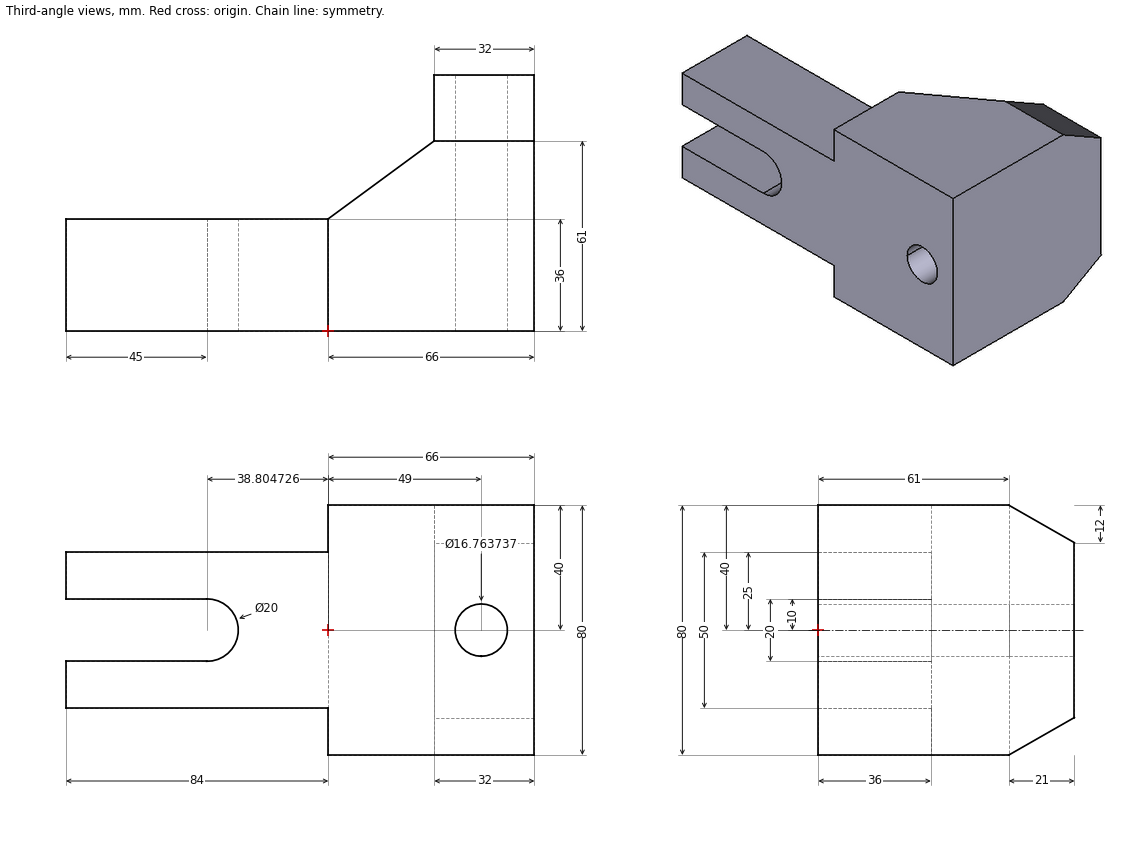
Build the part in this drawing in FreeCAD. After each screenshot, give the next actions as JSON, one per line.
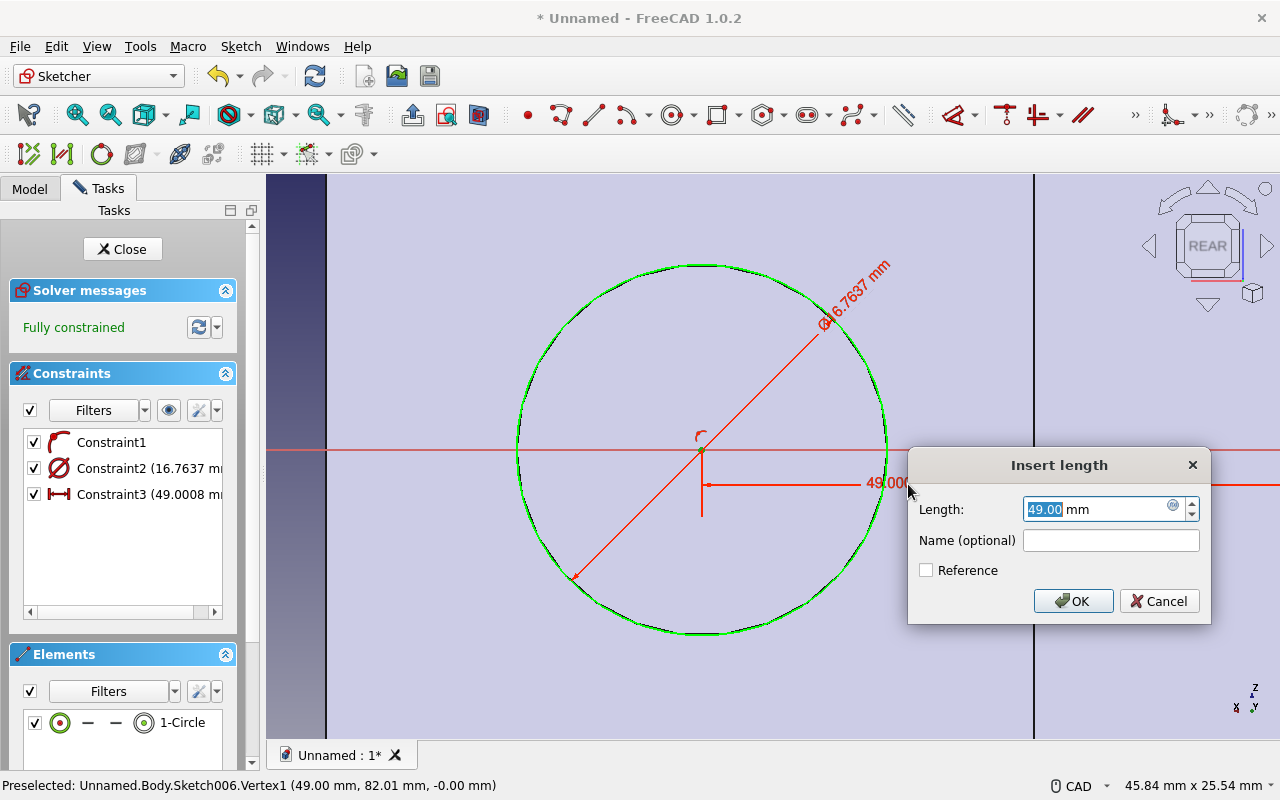
{"action": "type", "text": "49"}
{"action": "key", "text": "Return"}
{"action": "key", "text": "Escape"}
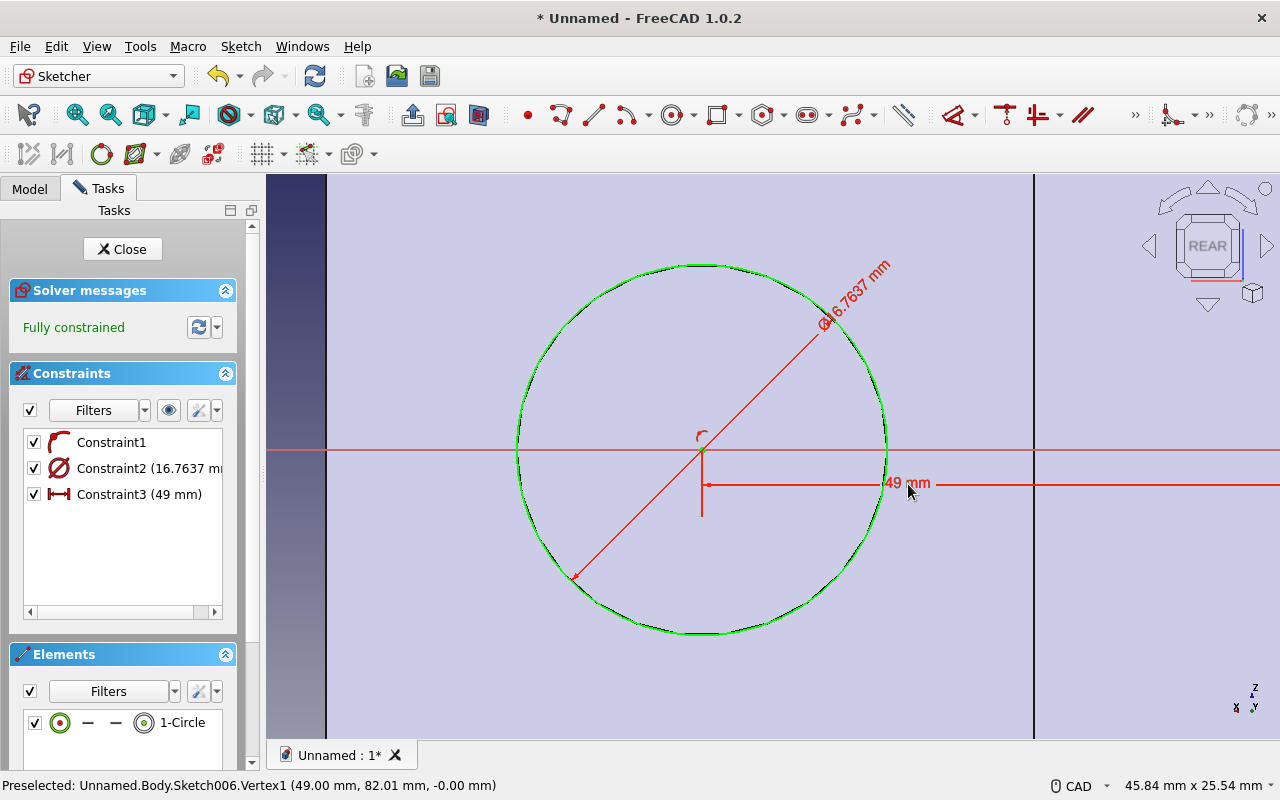
{"action": "left_click", "coordinate": [123, 249]}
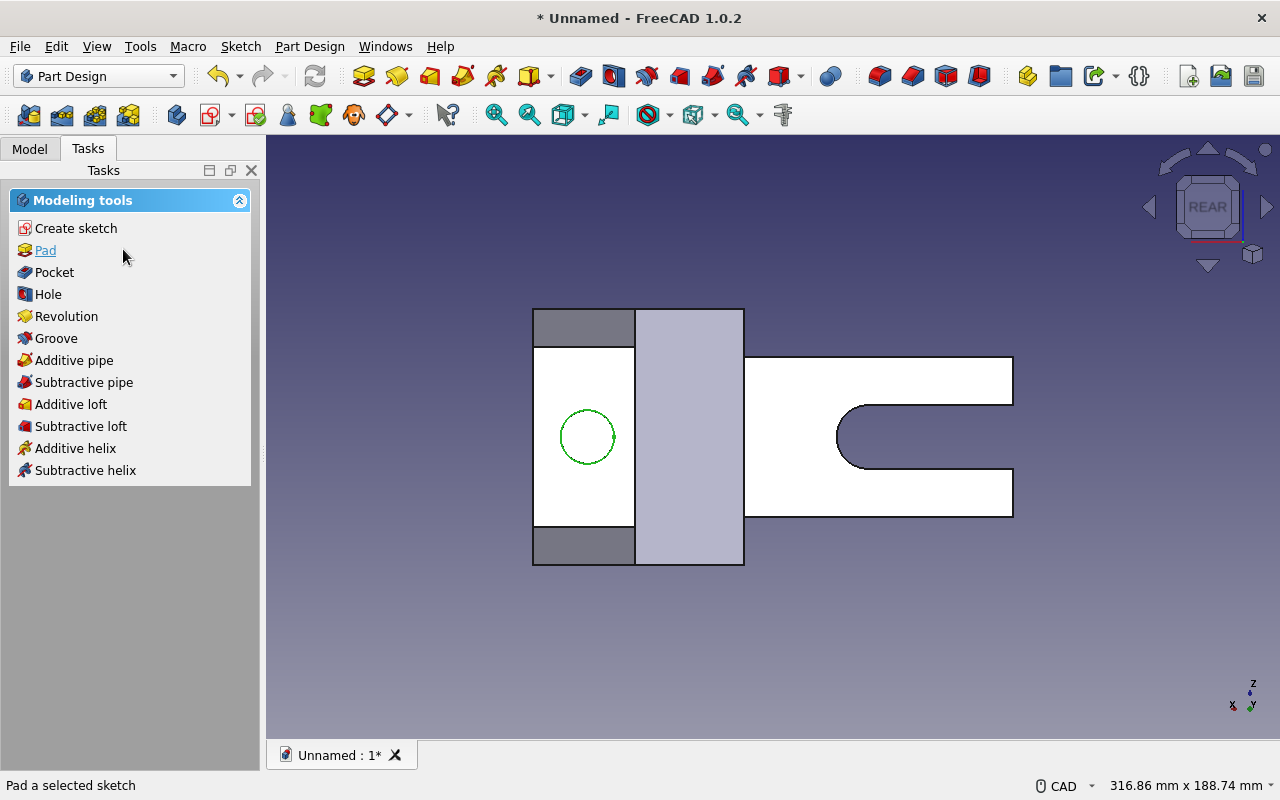
{"action": "left_click", "coordinate": [581, 76]}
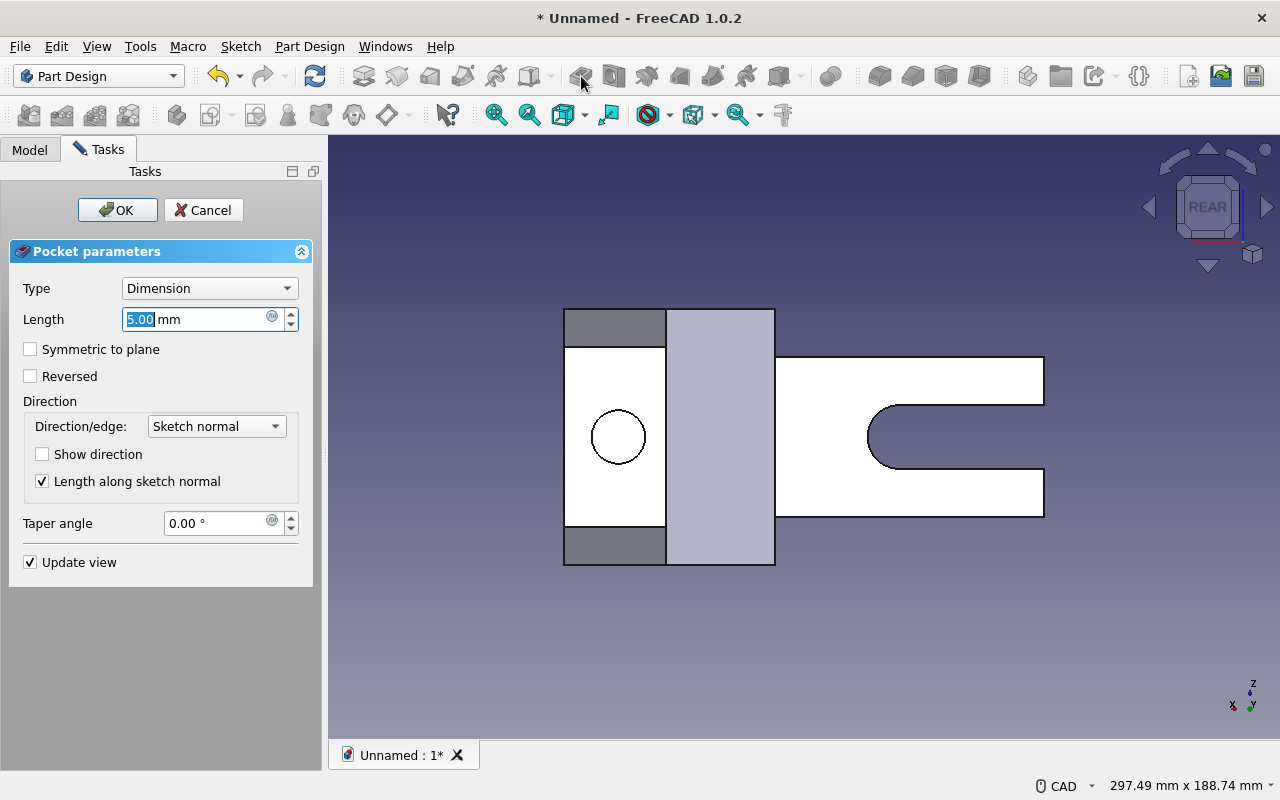
{"action": "left_click", "coordinate": [210, 288]}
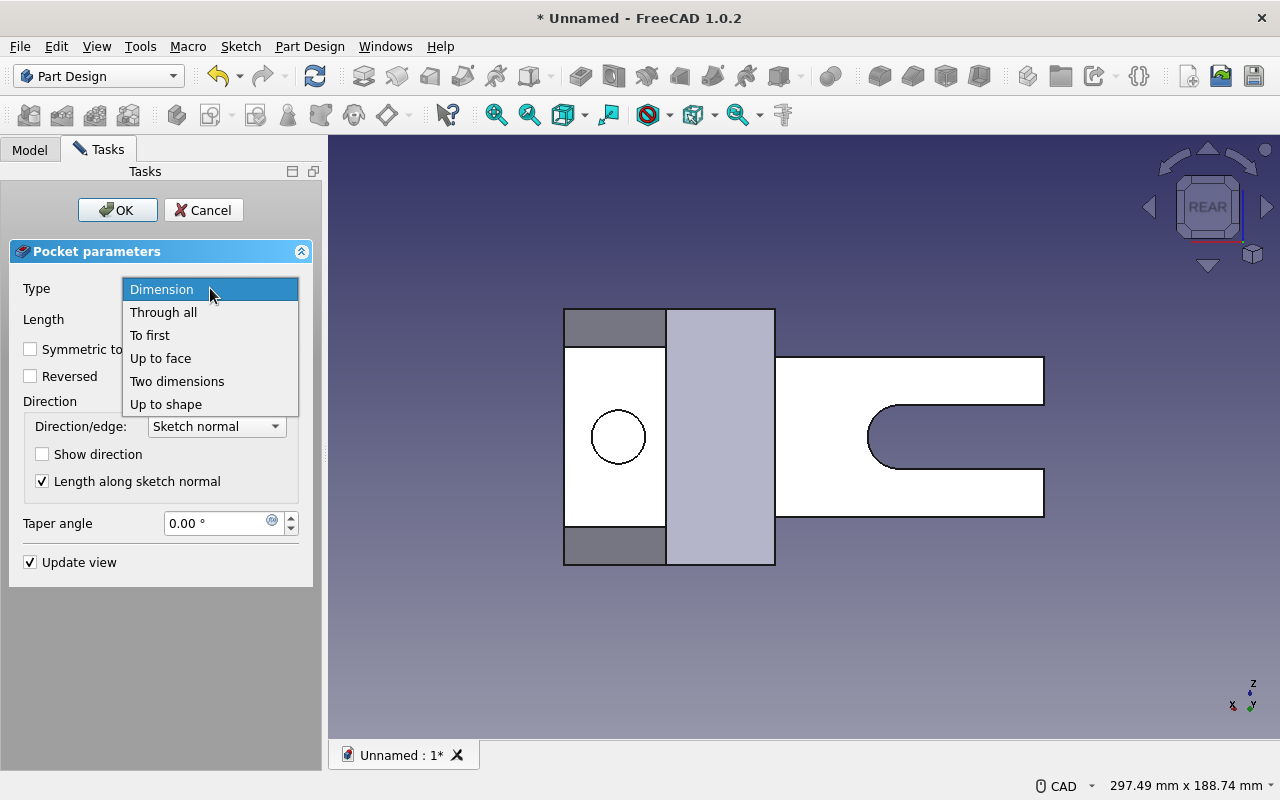
{"action": "left_click", "coordinate": [208, 312]}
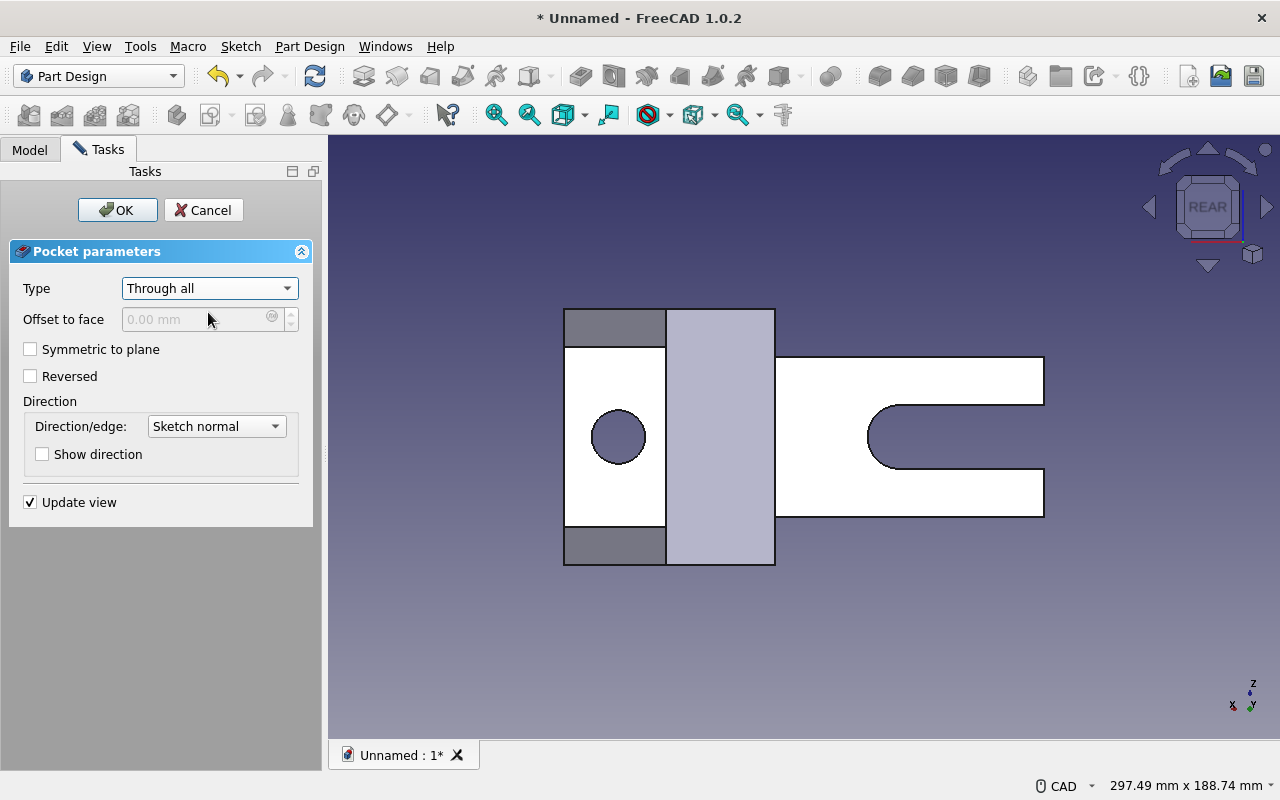
{"action": "left_click", "coordinate": [118, 210]}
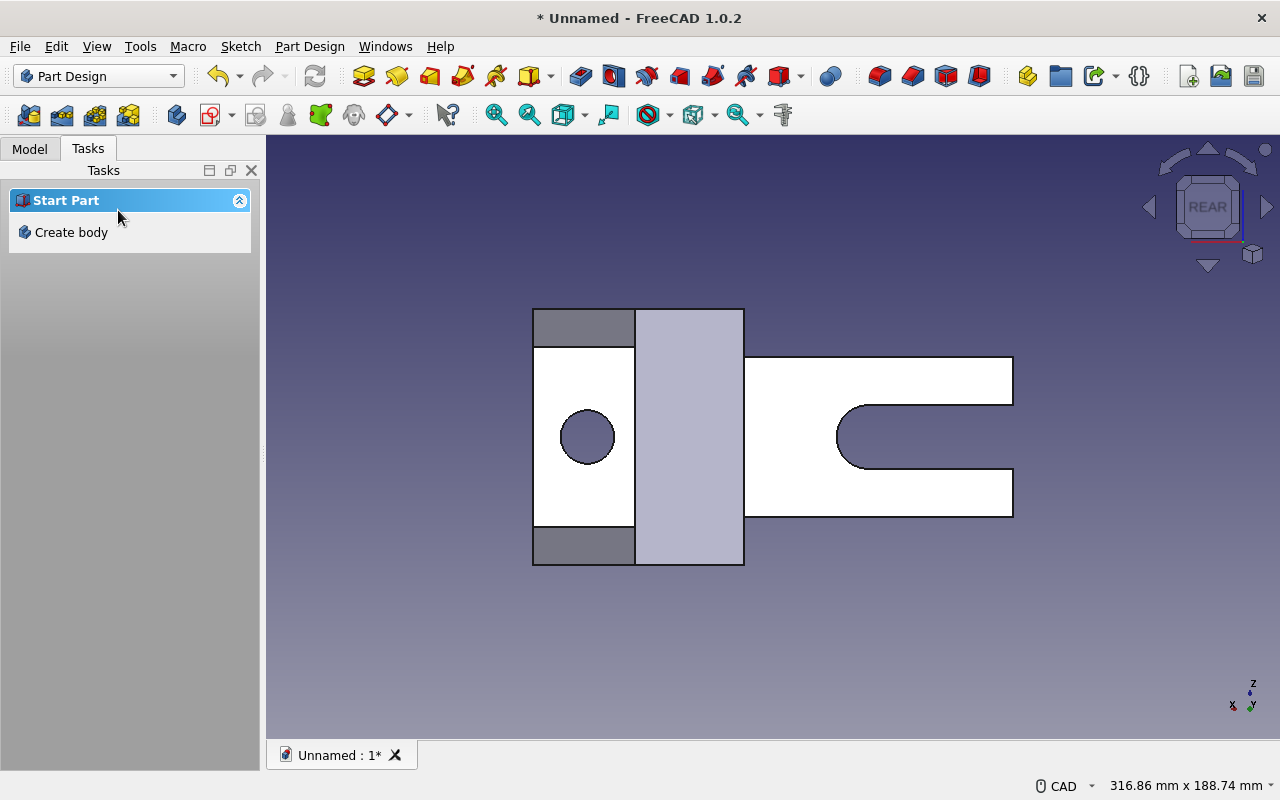
{"action": "key", "text": "0"}